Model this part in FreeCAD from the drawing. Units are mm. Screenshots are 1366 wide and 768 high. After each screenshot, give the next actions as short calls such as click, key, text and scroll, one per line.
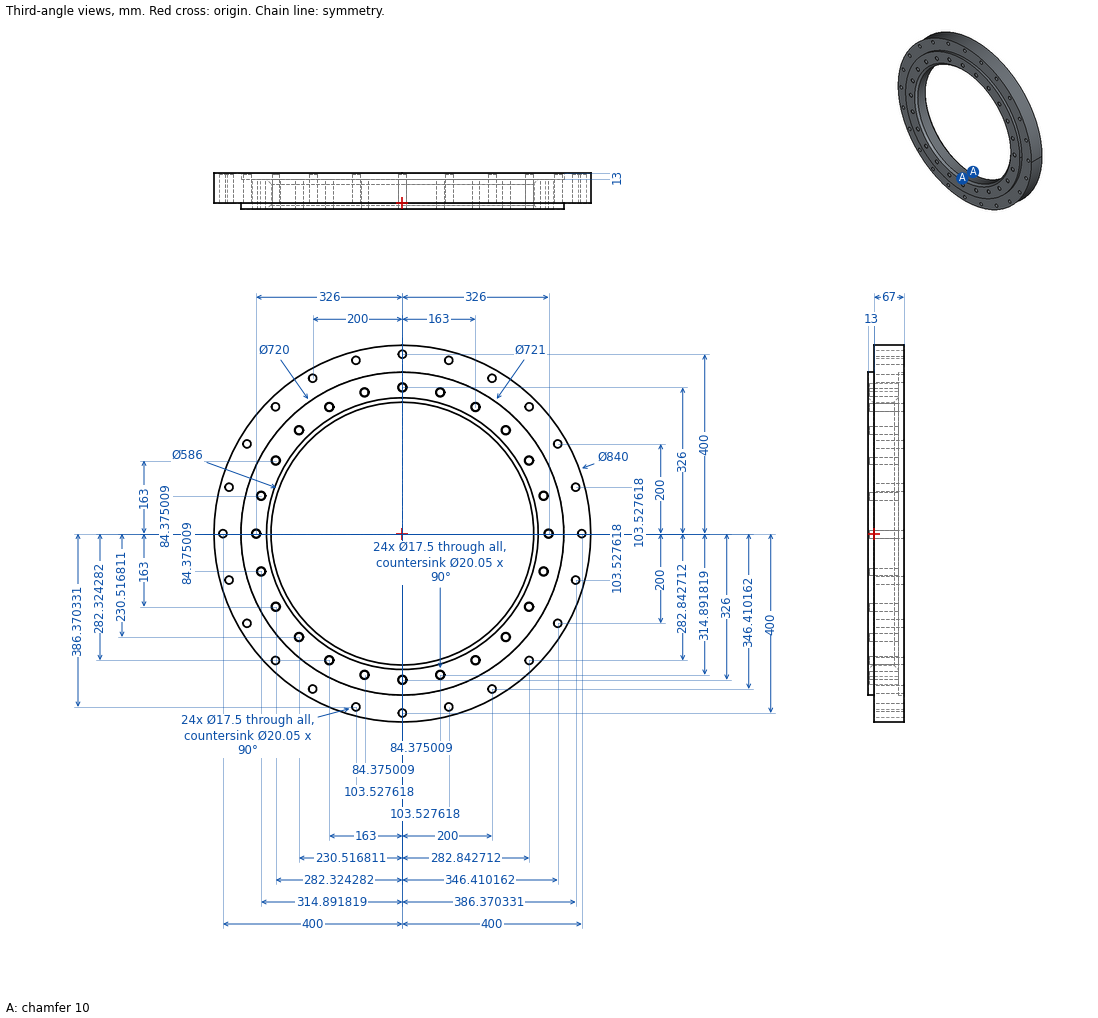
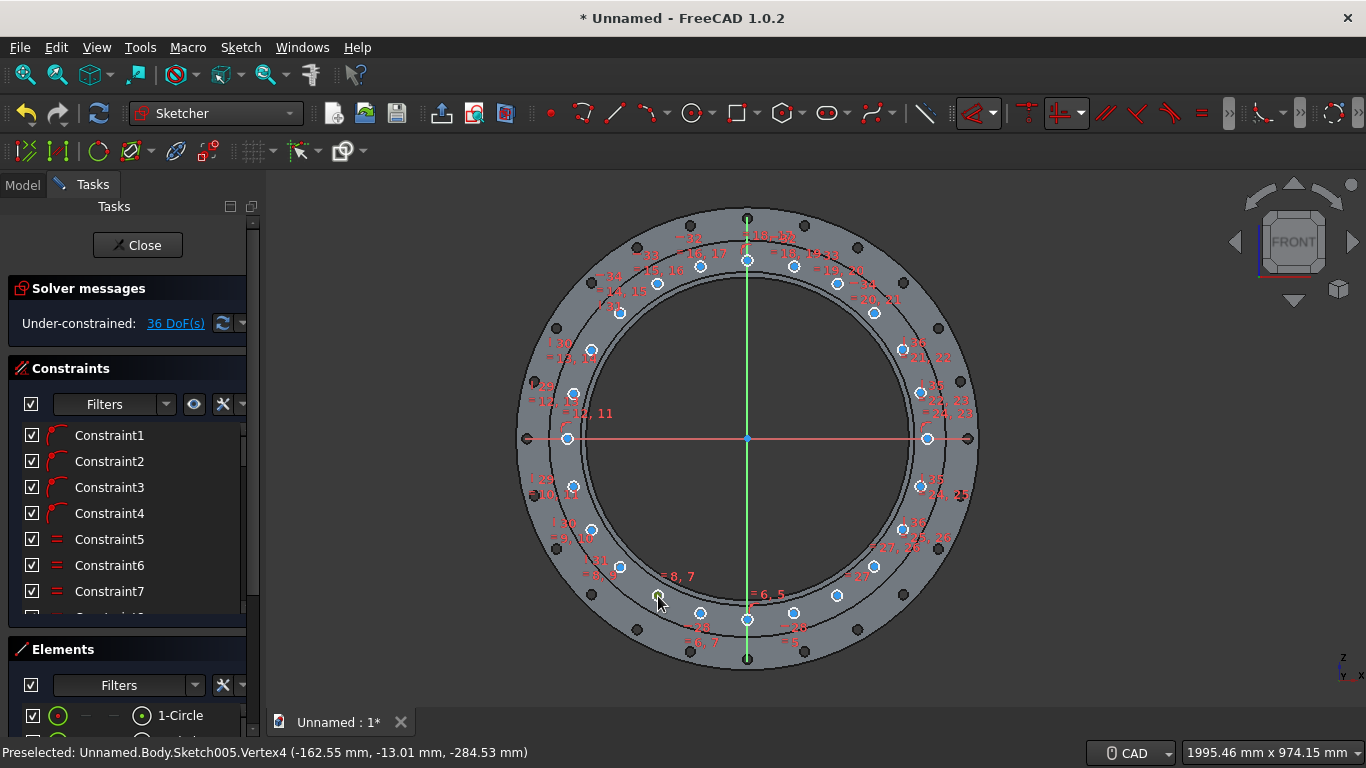
click(658, 284)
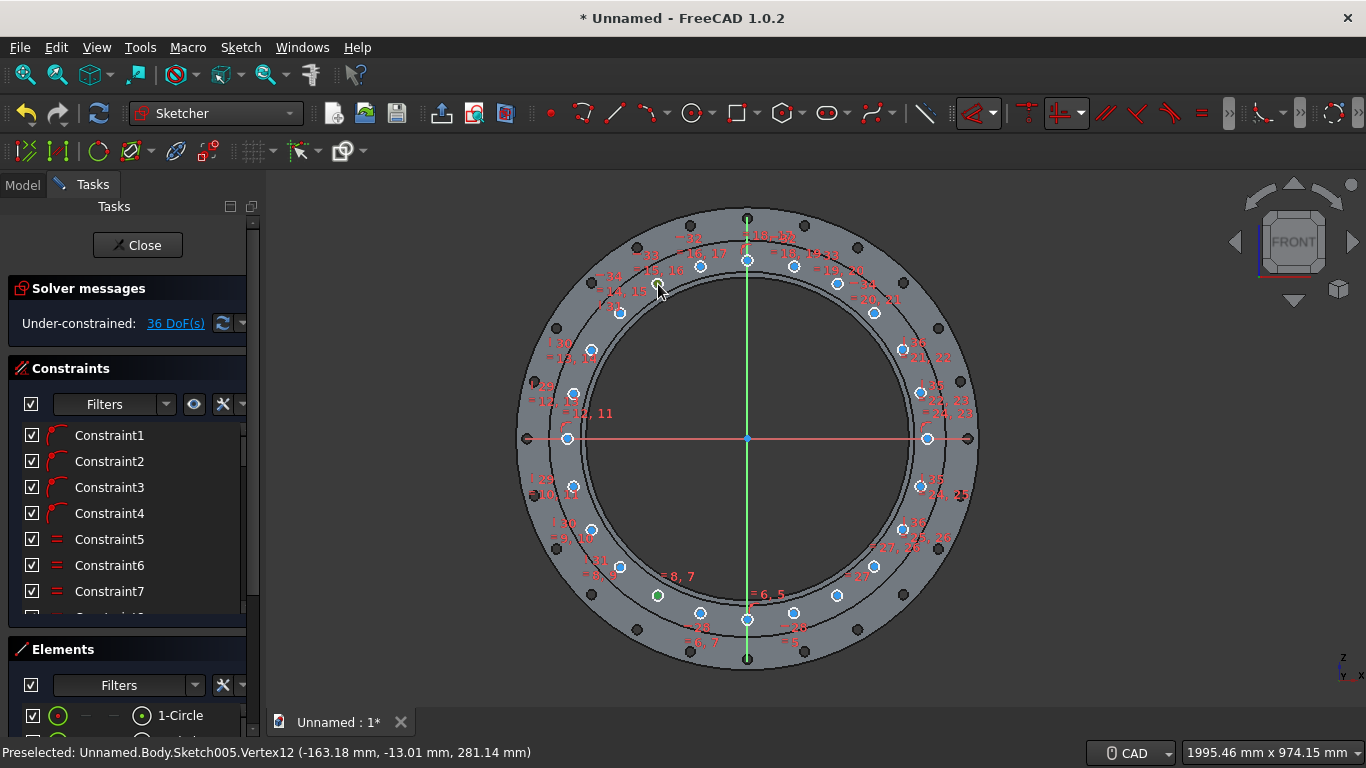
click(618, 439)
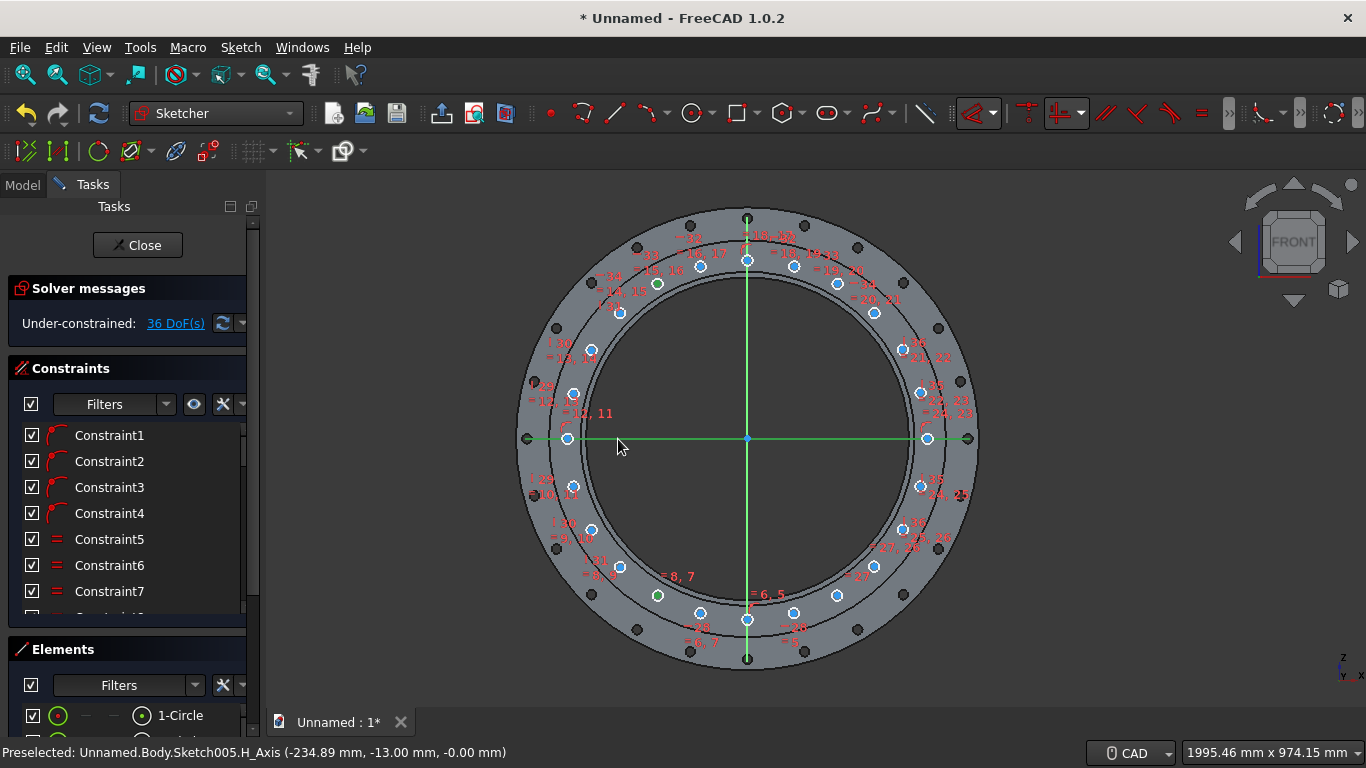
key(s)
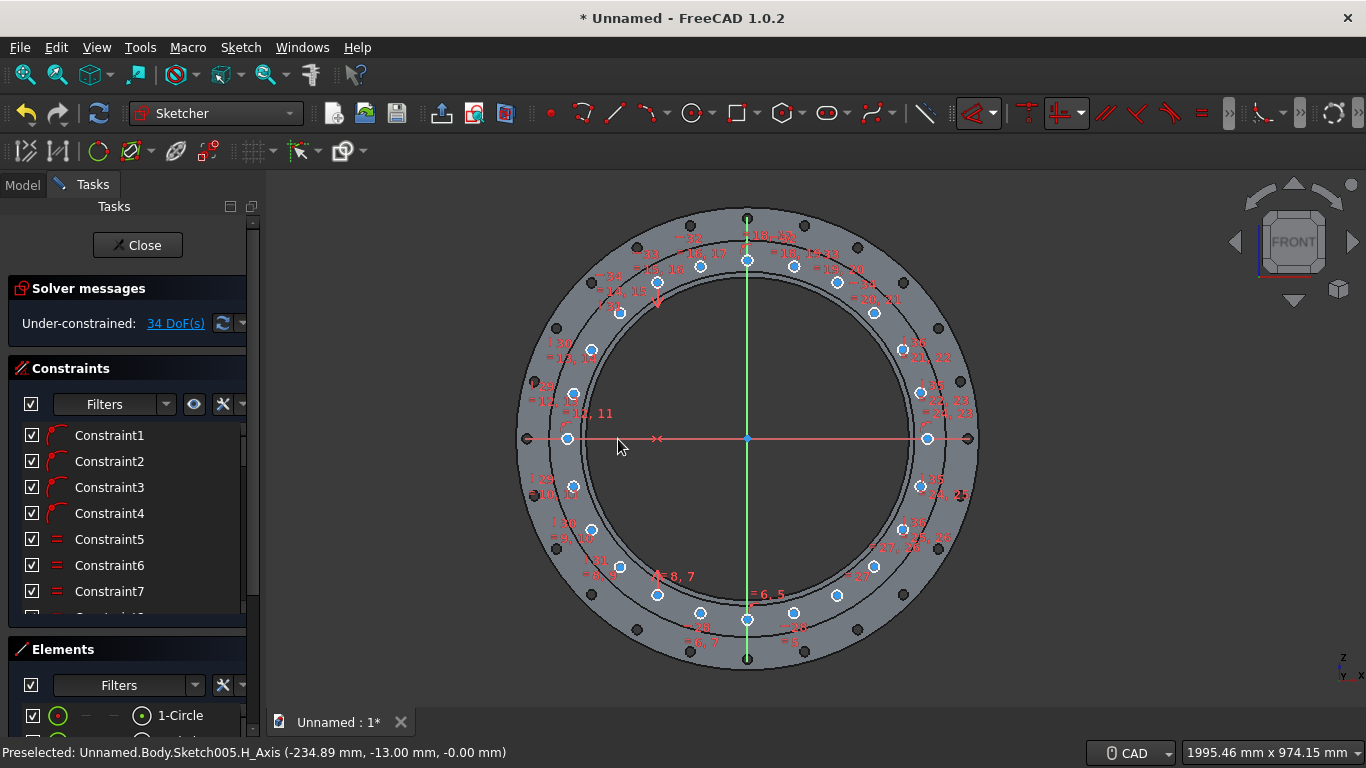
click(701, 613)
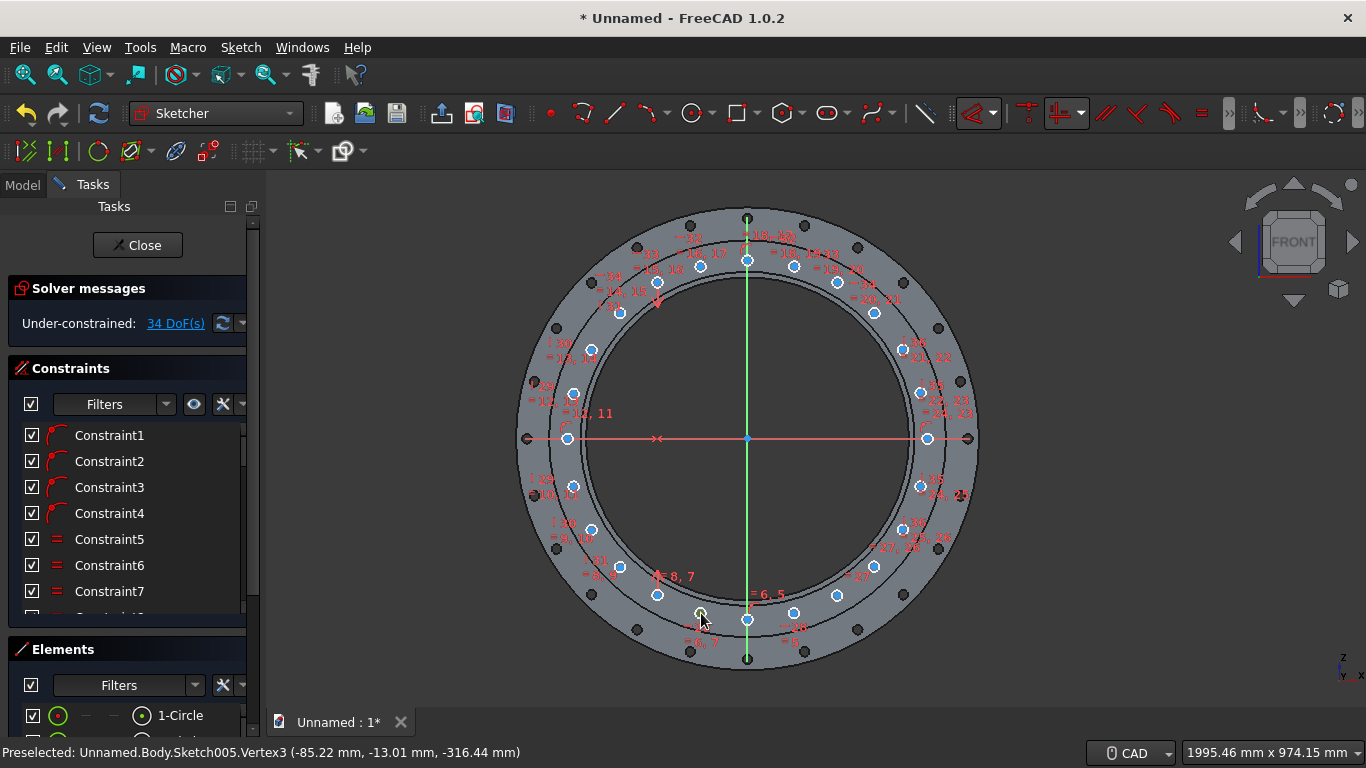
click(701, 267)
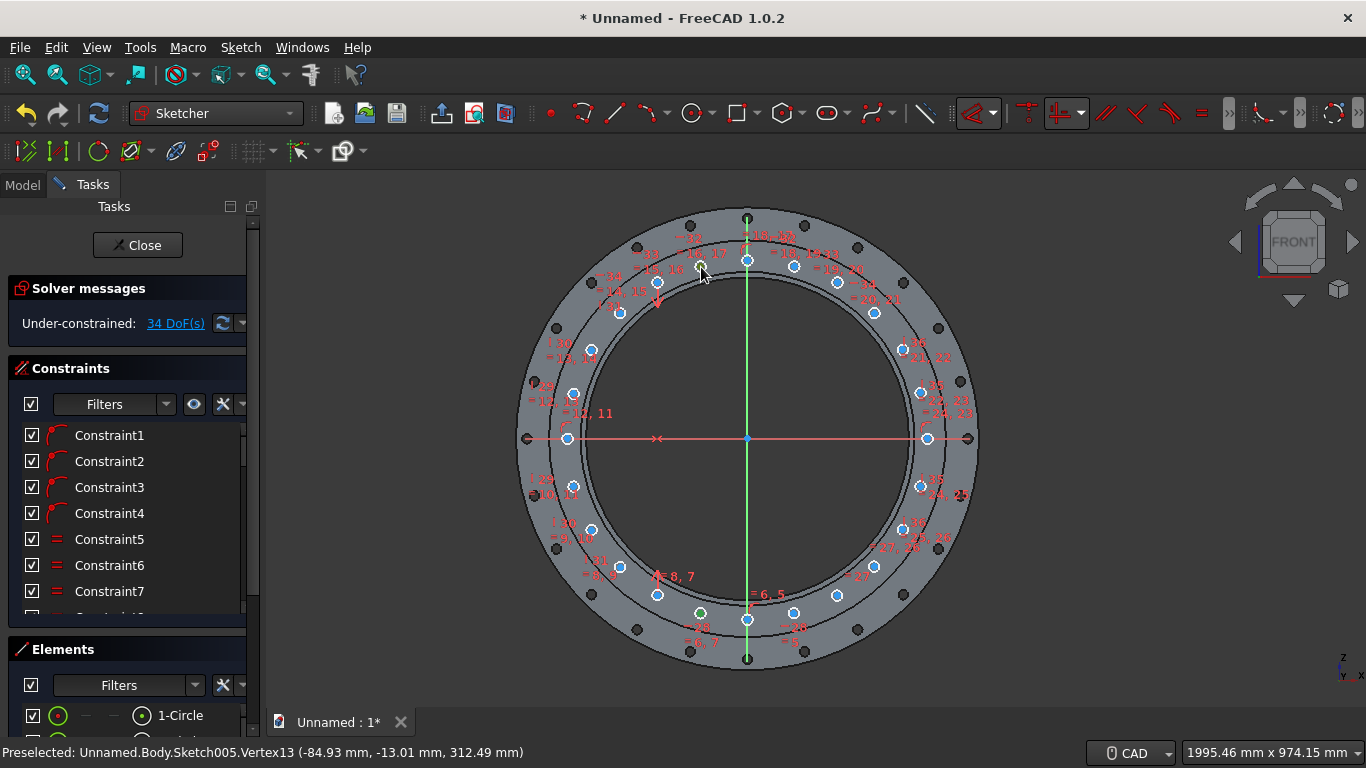
click(618, 439)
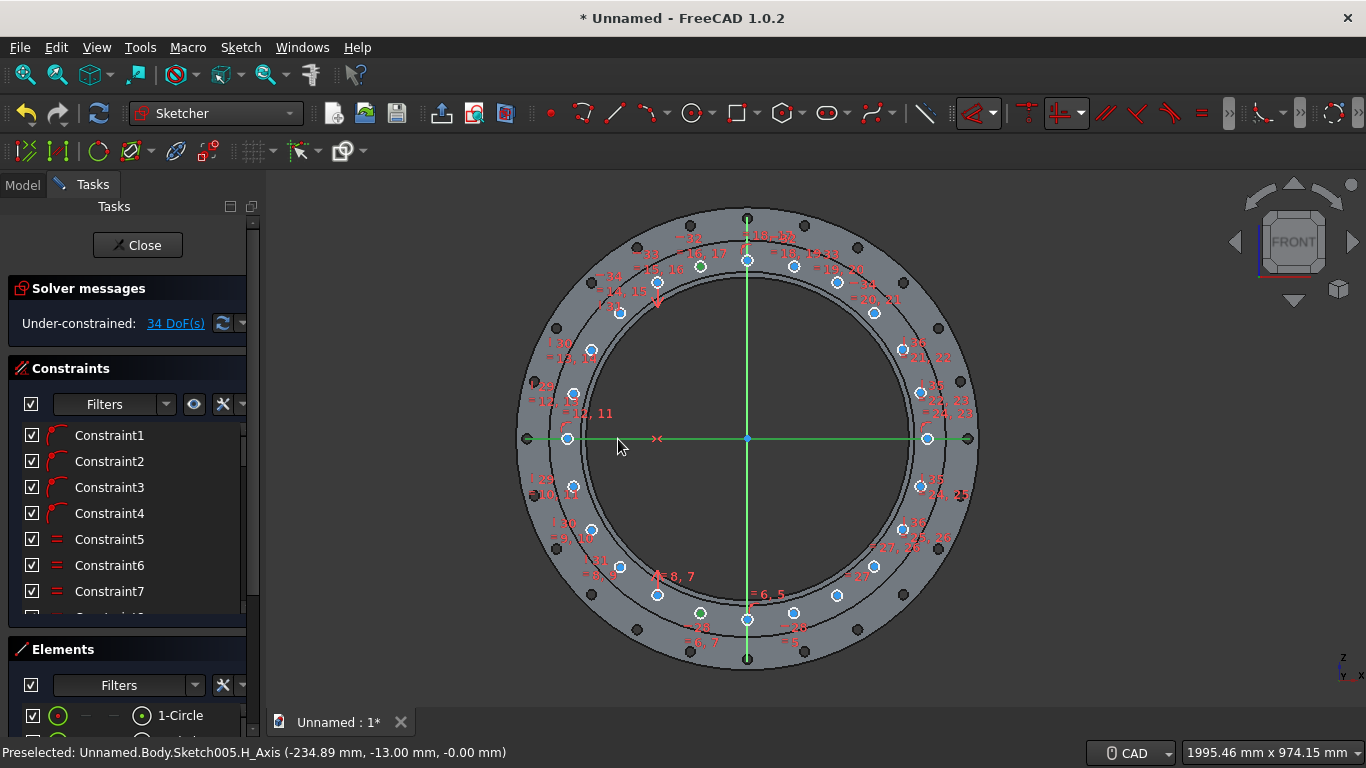
key(s)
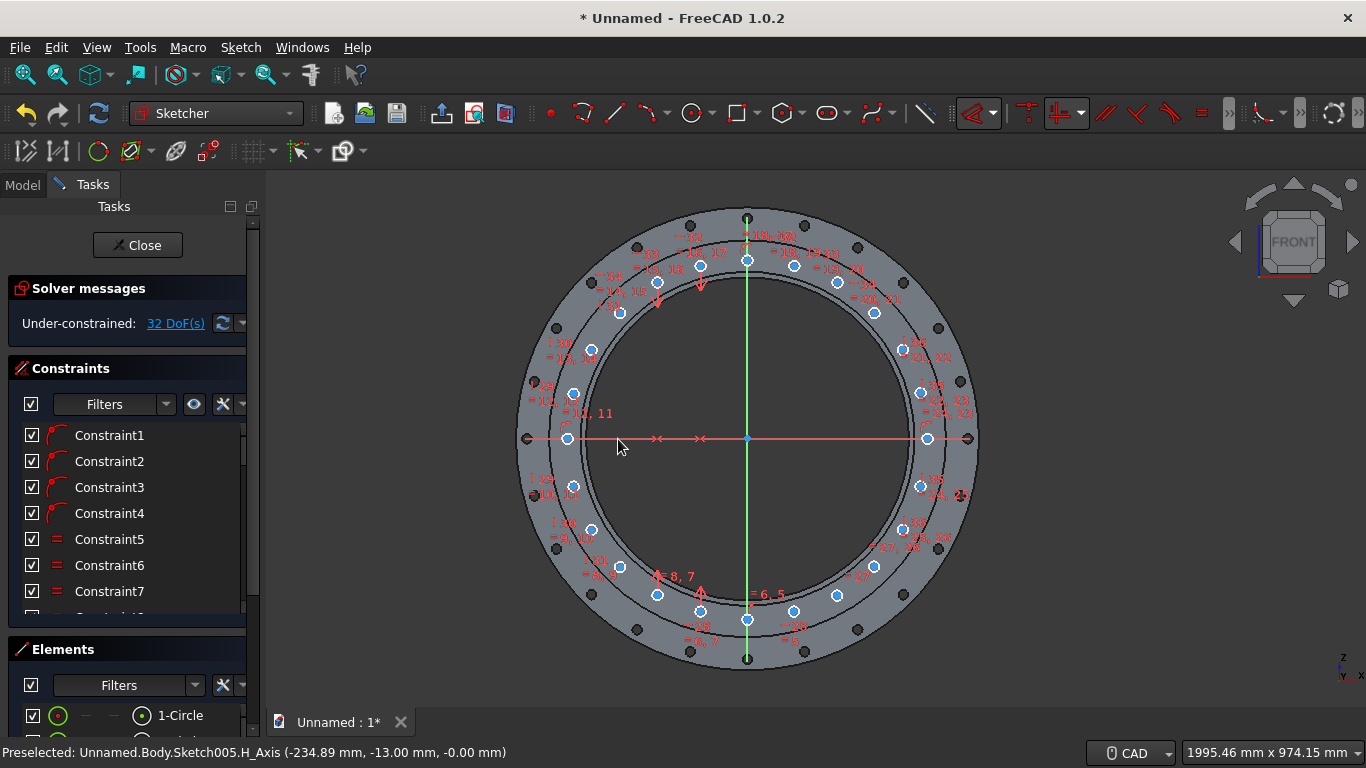
scroll(592, 350, up, 4)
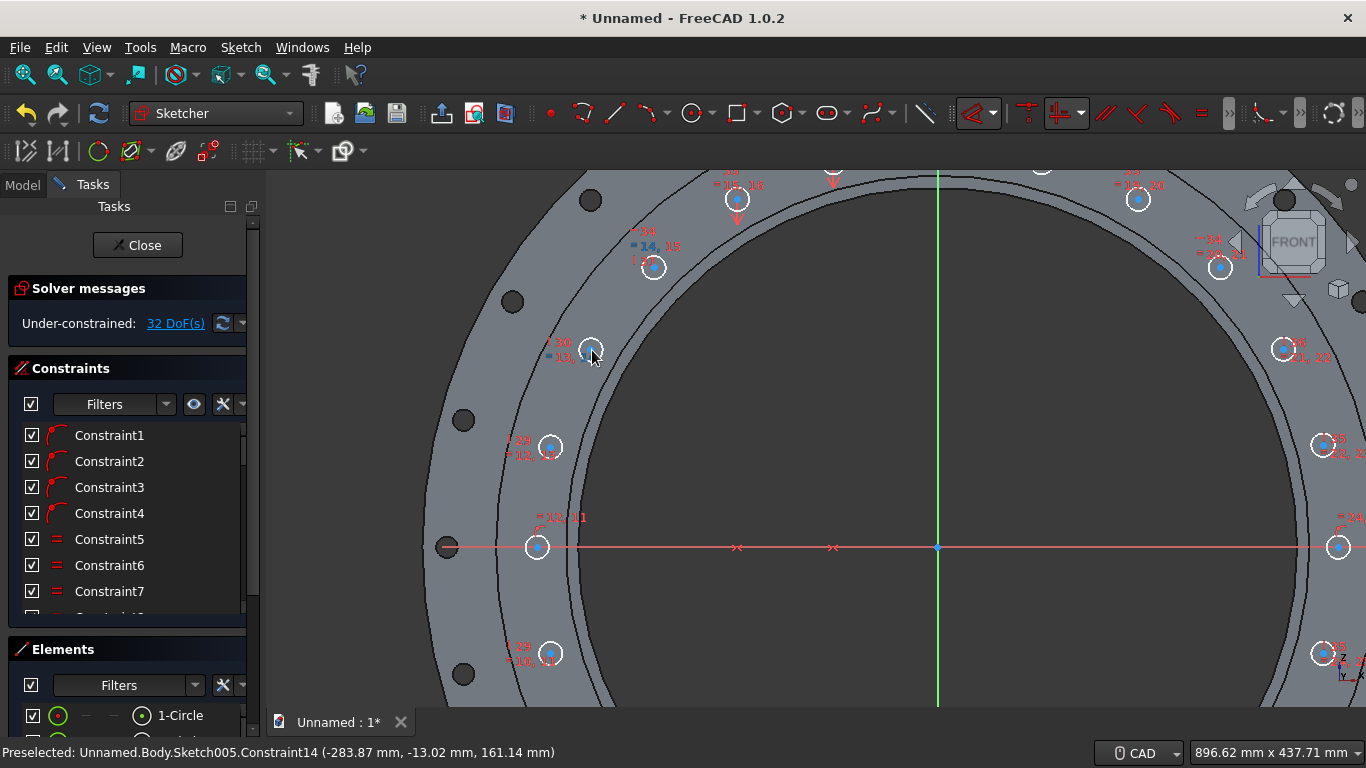
scroll(591, 350, up, 4)